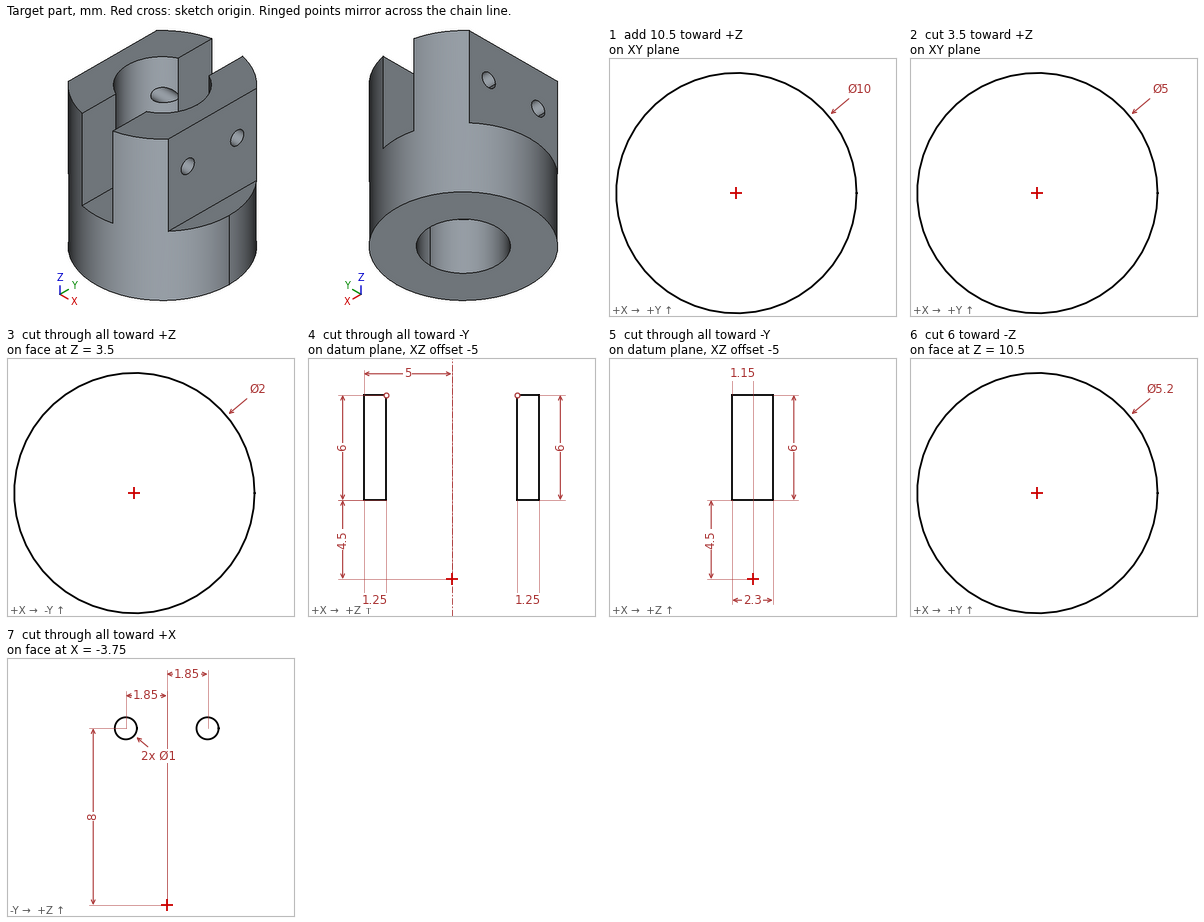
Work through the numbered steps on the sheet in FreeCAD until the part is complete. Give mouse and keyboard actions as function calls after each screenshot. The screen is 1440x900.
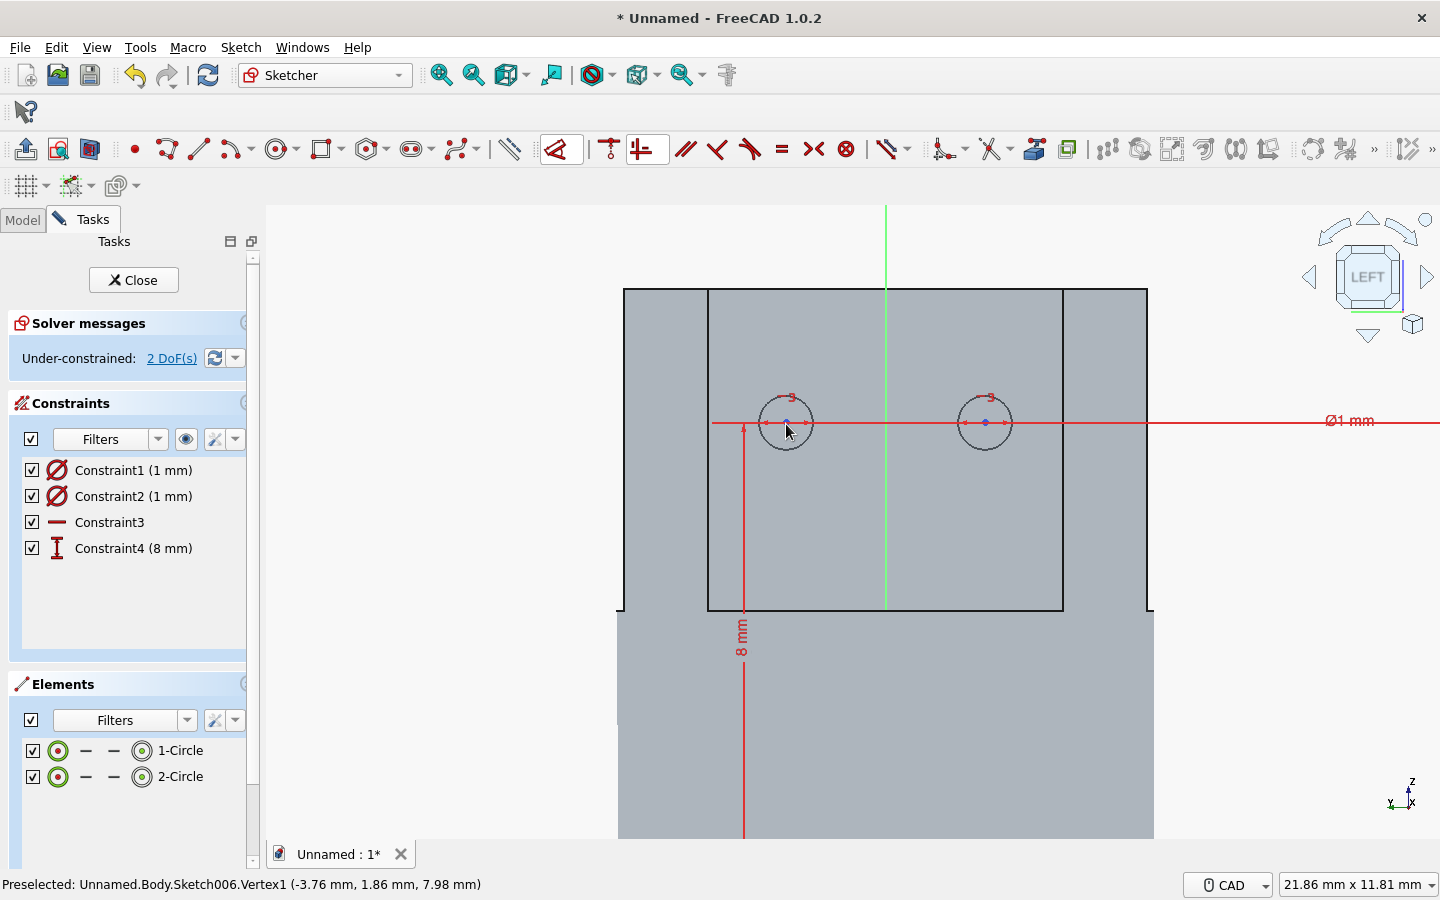
click(786, 423)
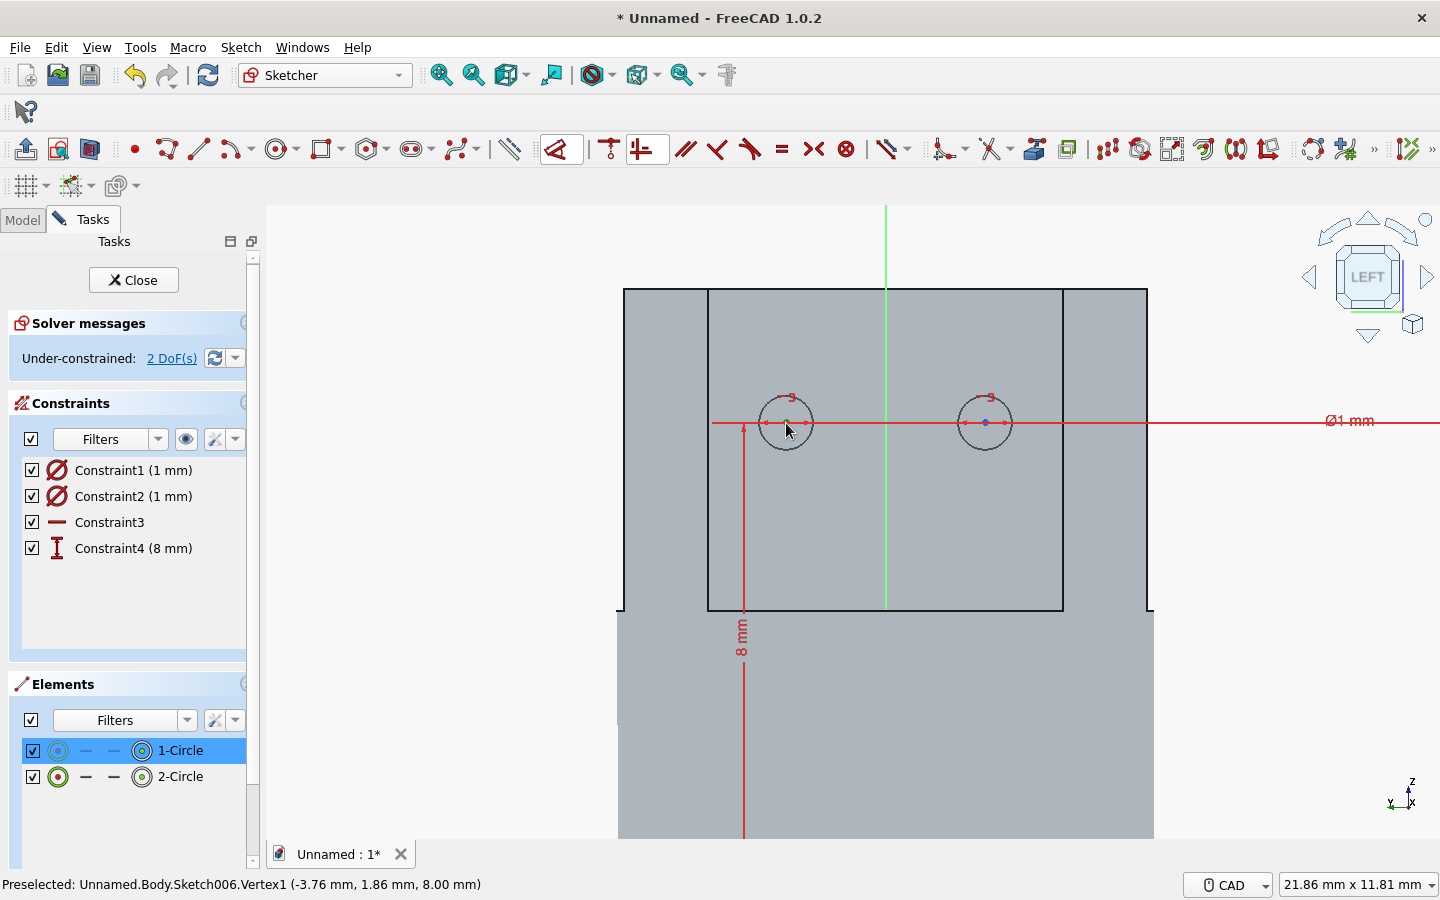
key(l)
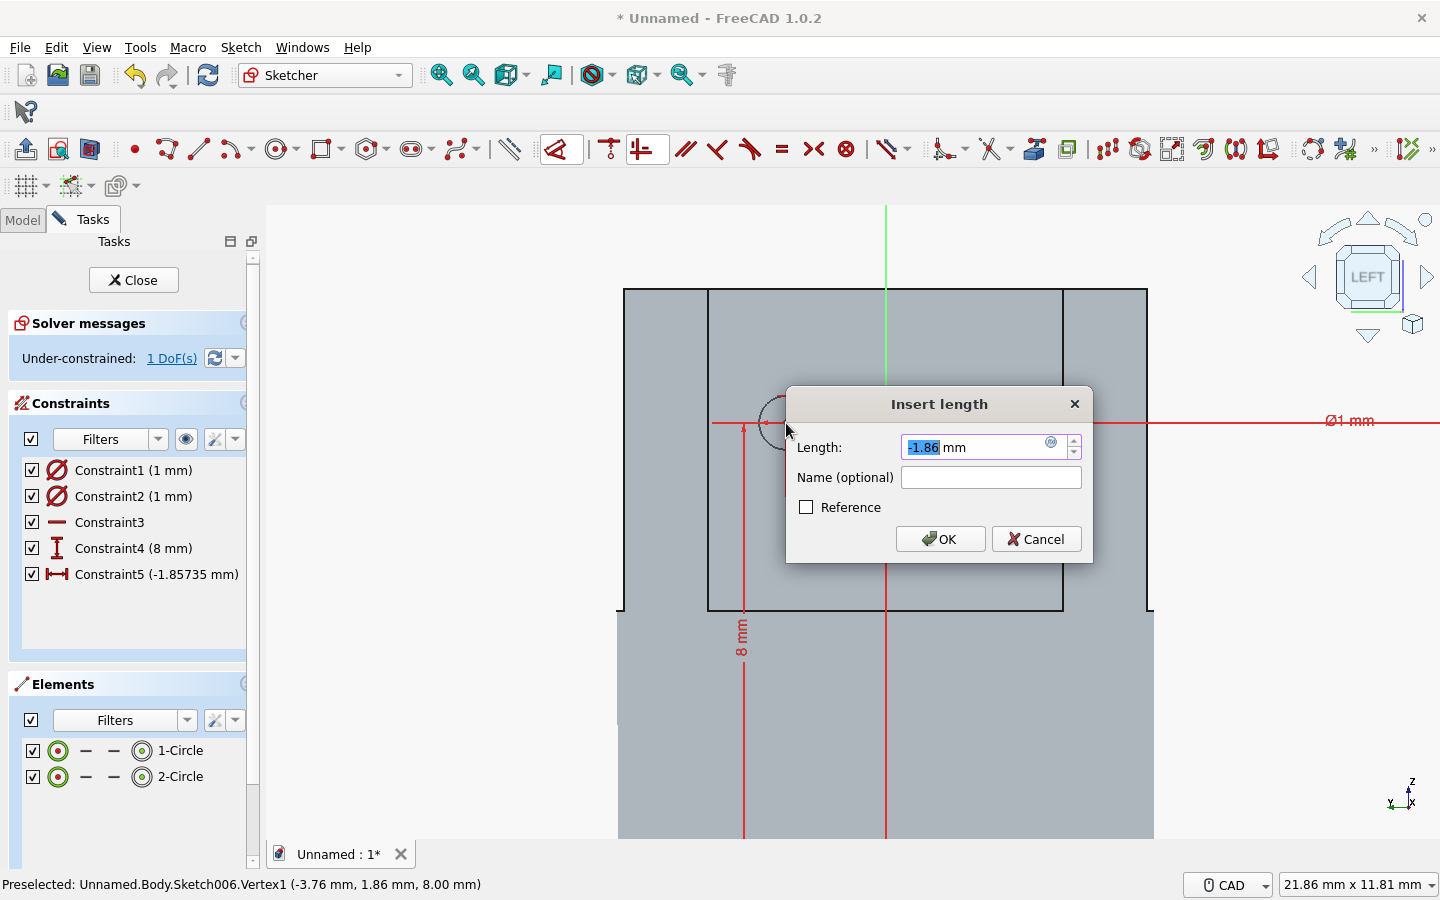
text(-1.85)
key(Return)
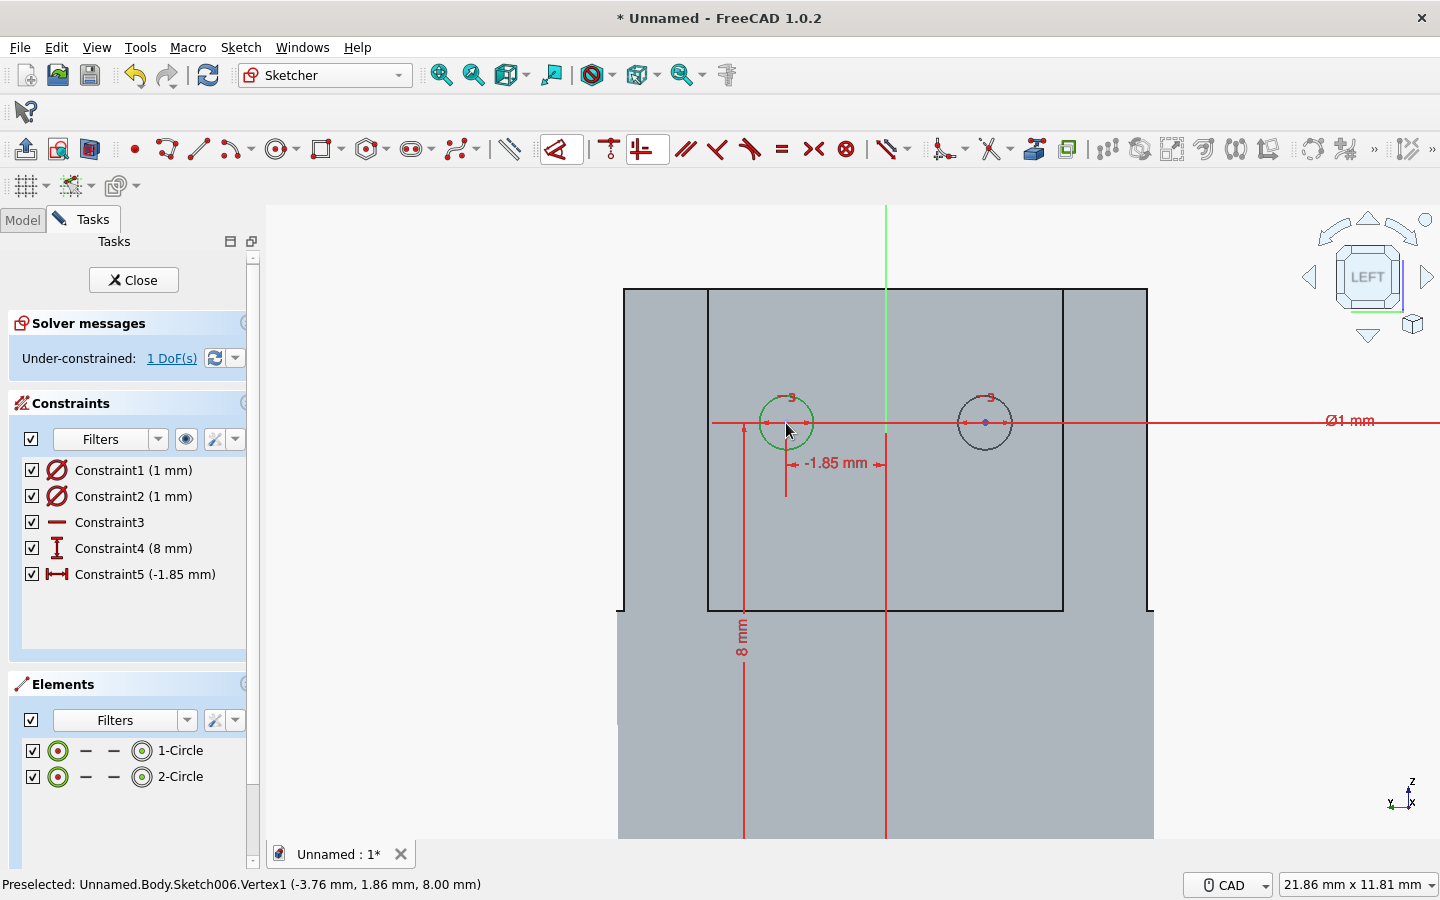
click(985, 423)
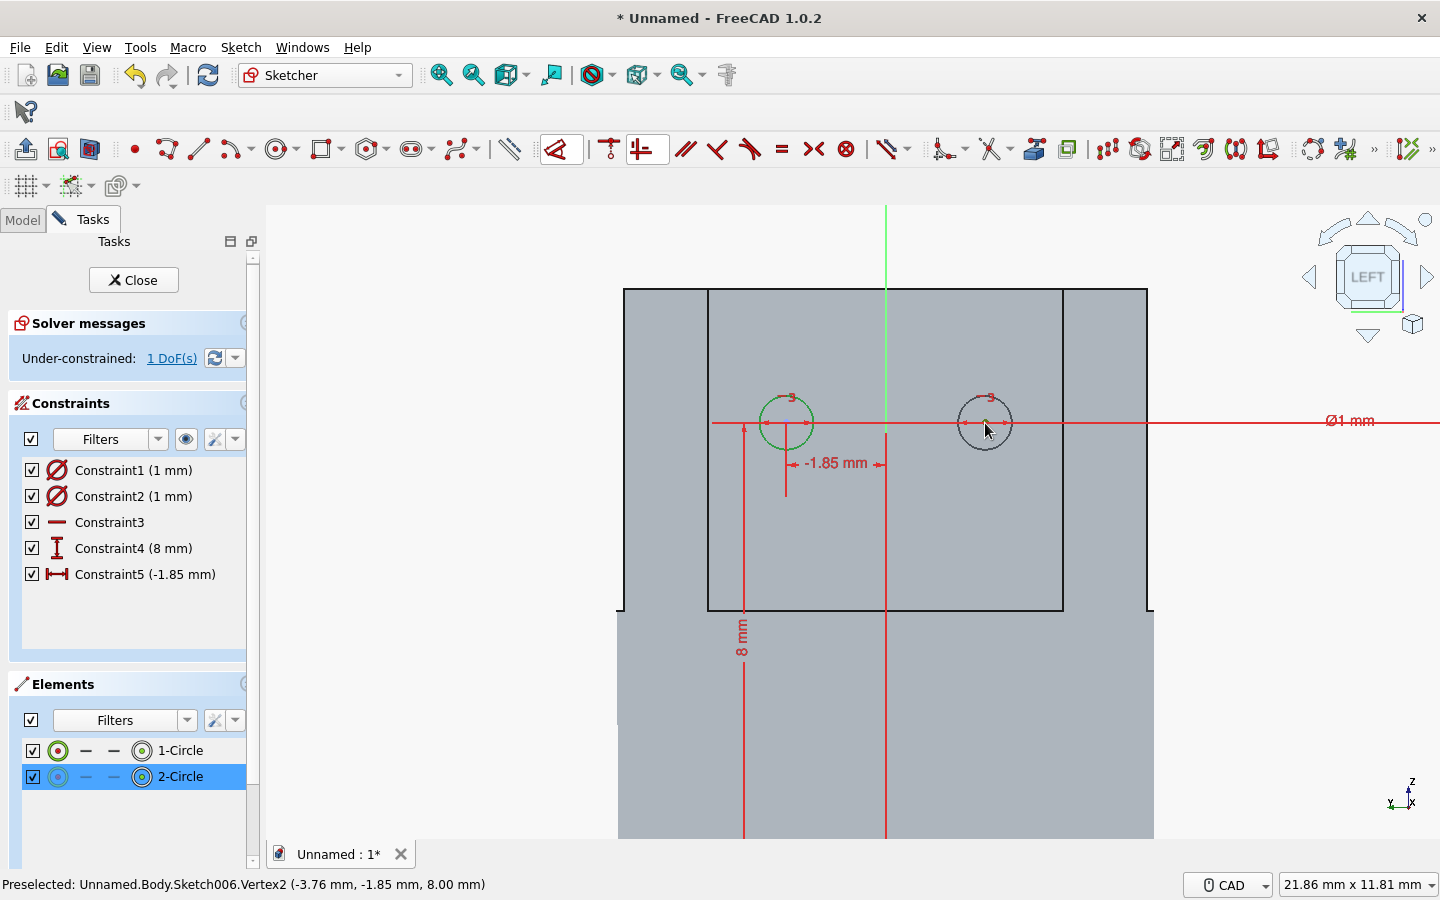
key(l)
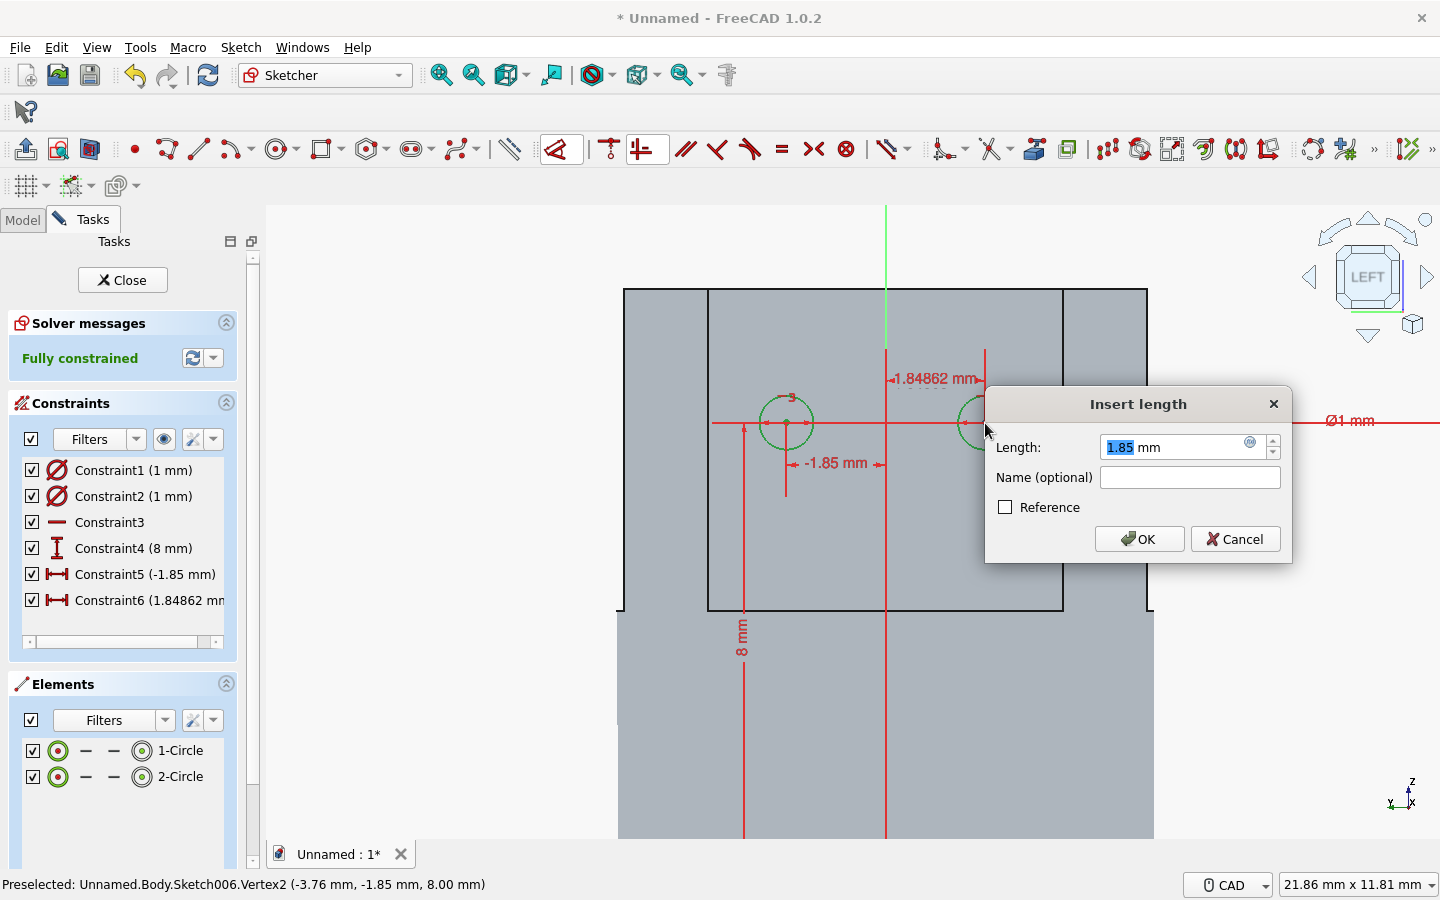
text(1.85)
key(Return)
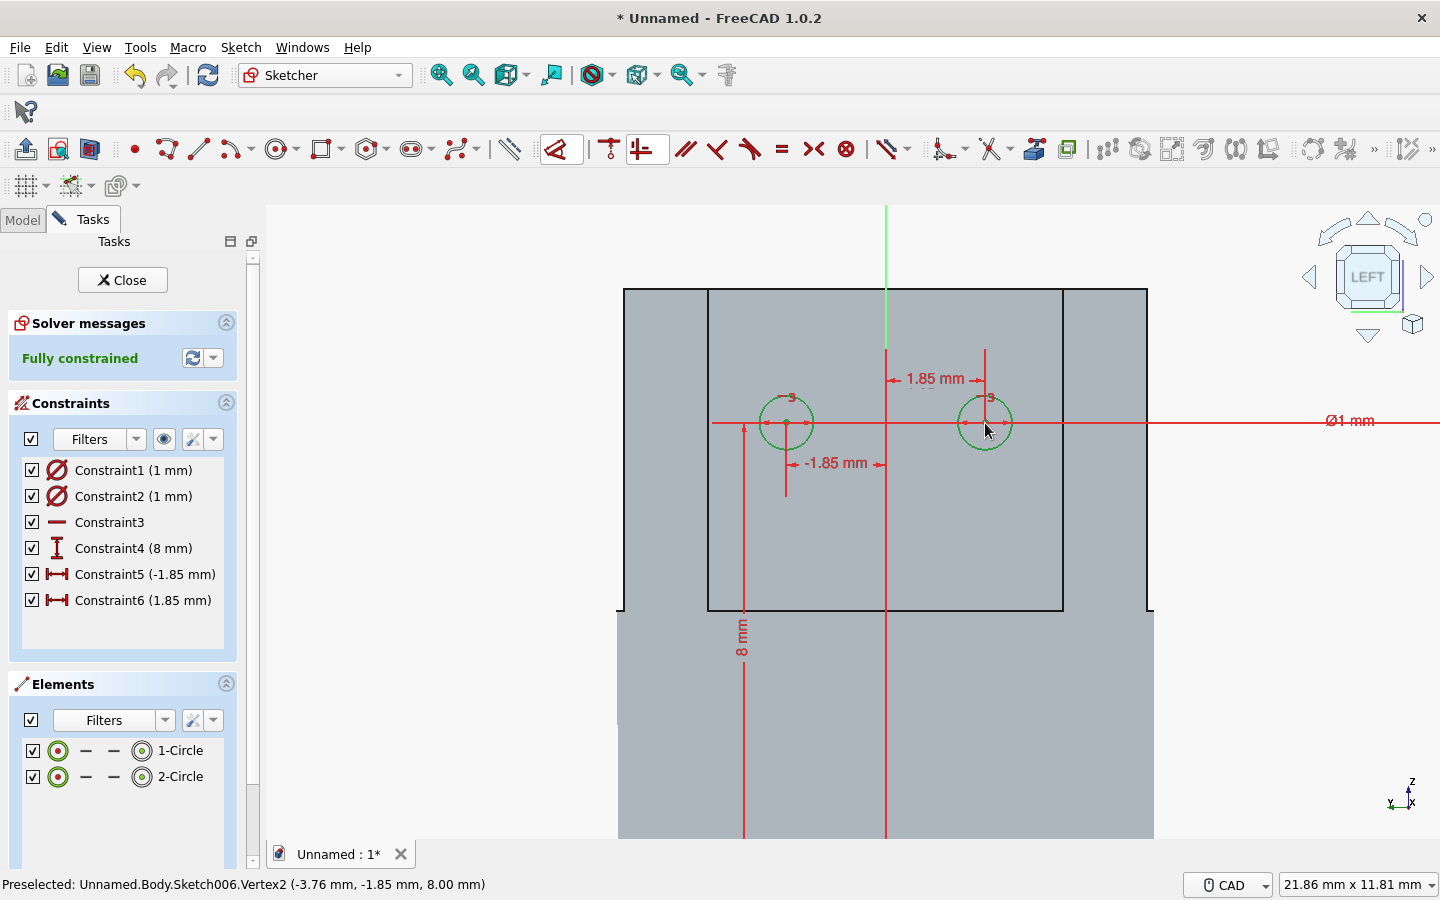
click(123, 280)